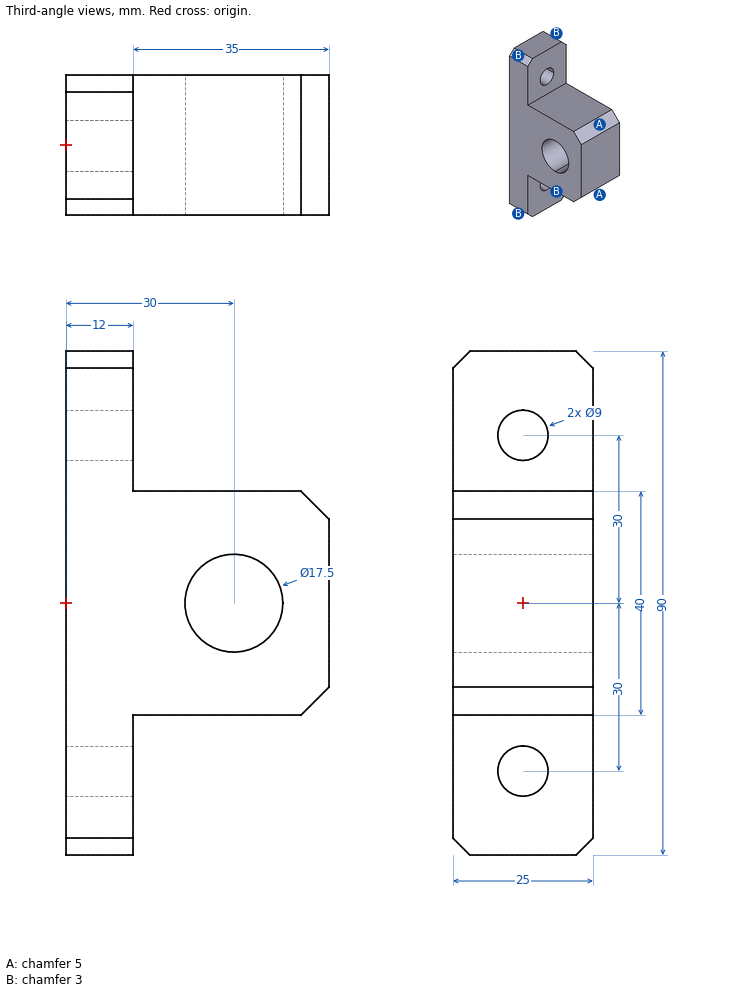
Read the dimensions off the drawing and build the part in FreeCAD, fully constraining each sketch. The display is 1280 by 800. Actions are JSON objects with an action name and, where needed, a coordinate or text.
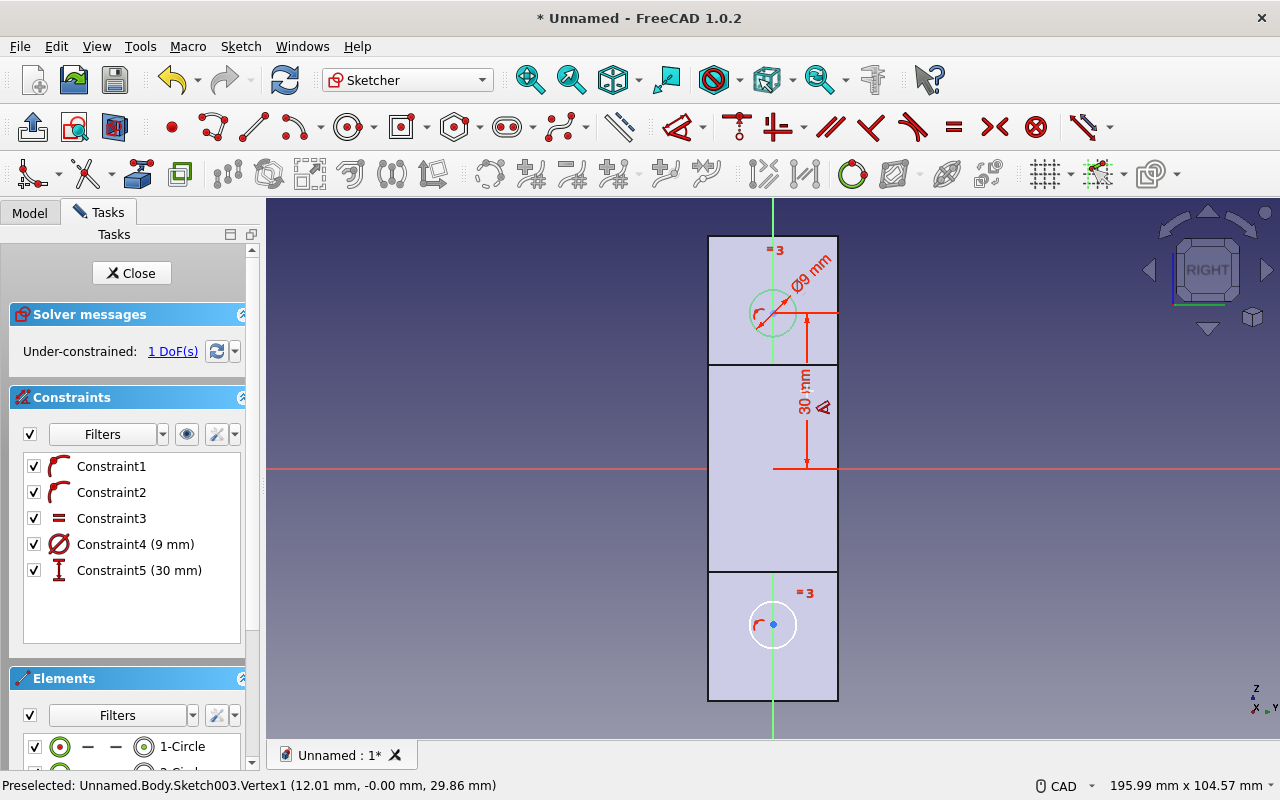
{"action": "left_click", "coordinate": [773, 625]}
{"action": "left_click", "coordinate": [807, 547]}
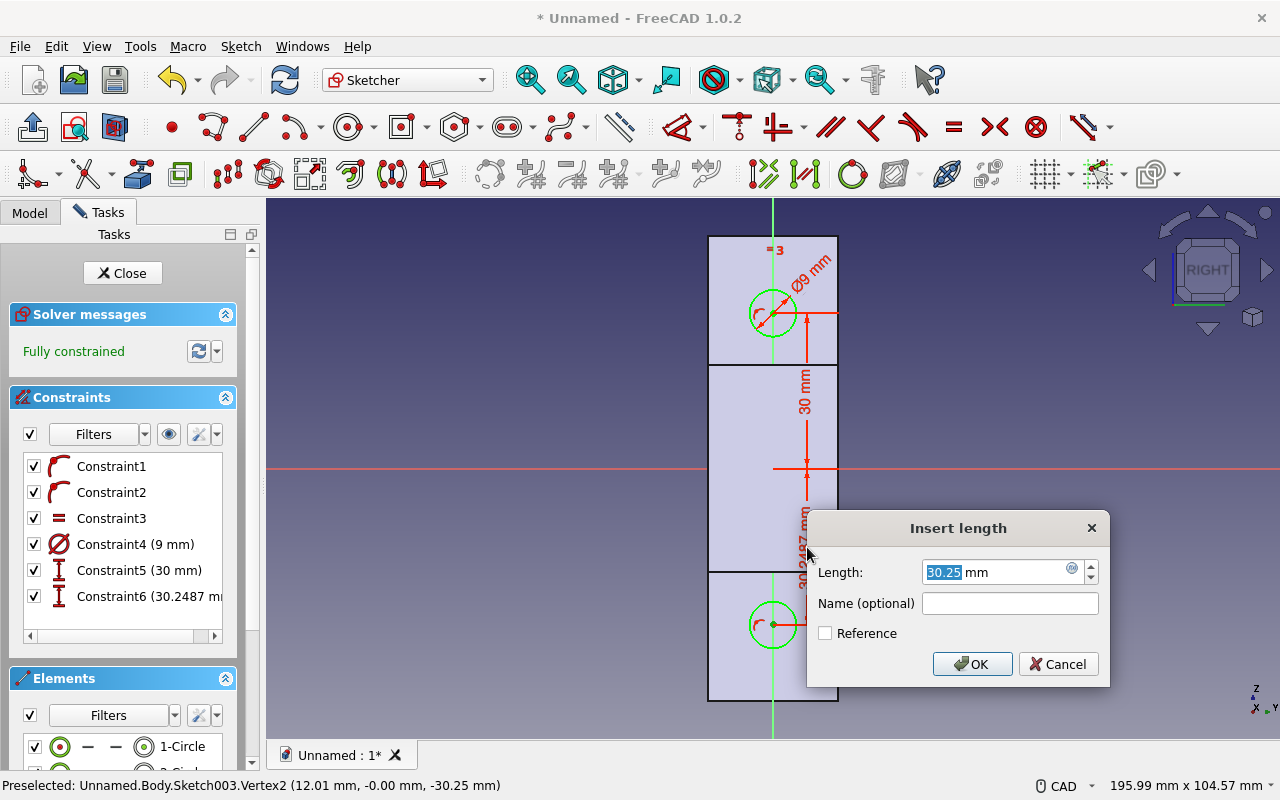
{"action": "type", "text": "30"}
{"action": "key", "text": "Return"}
{"action": "key", "text": "Escape"}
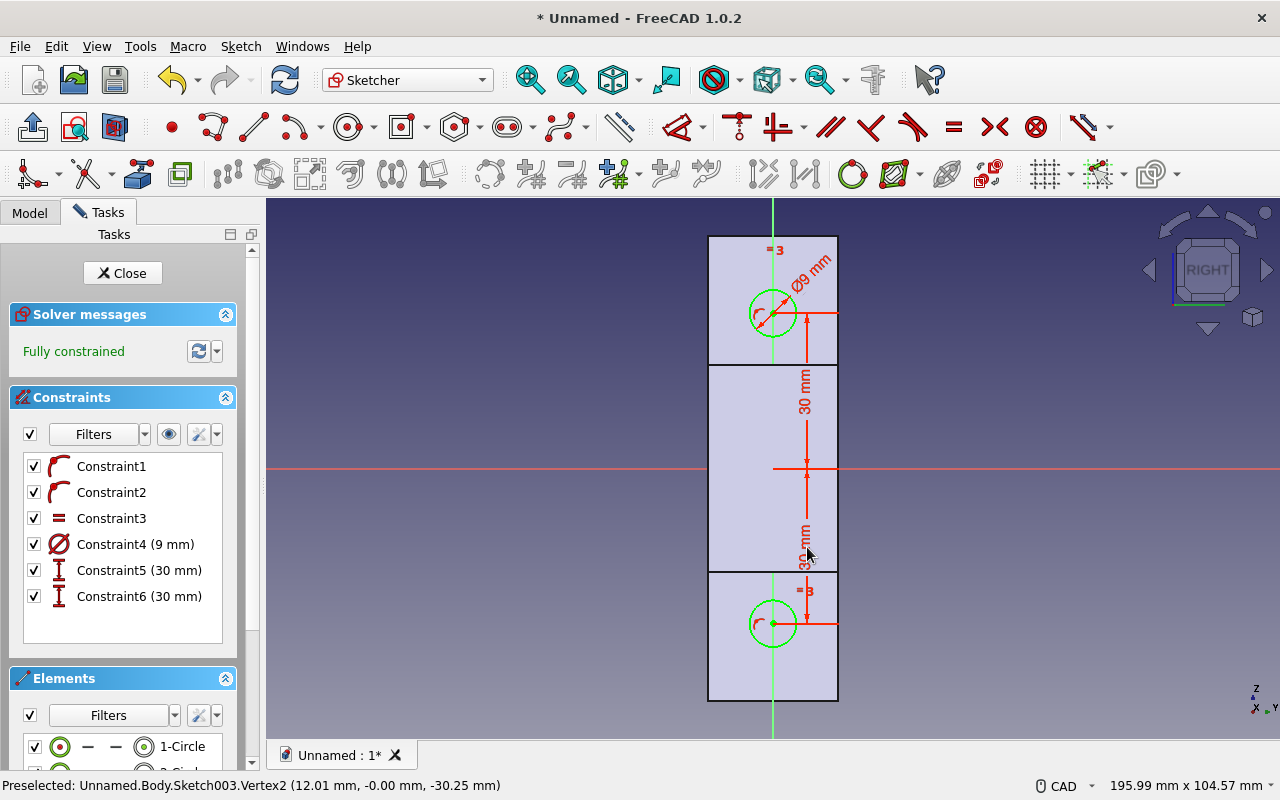
{"action": "left_click", "coordinate": [123, 273]}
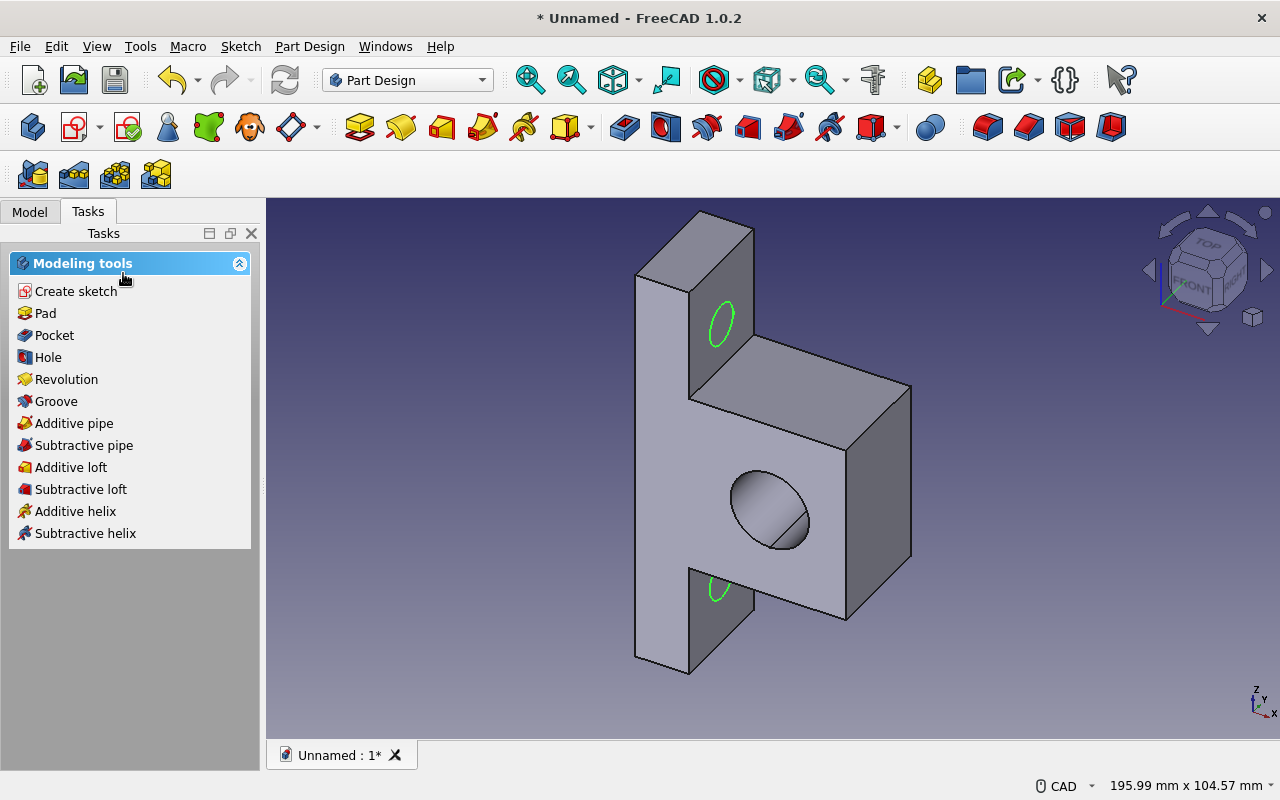
{"action": "left_click", "coordinate": [625, 128]}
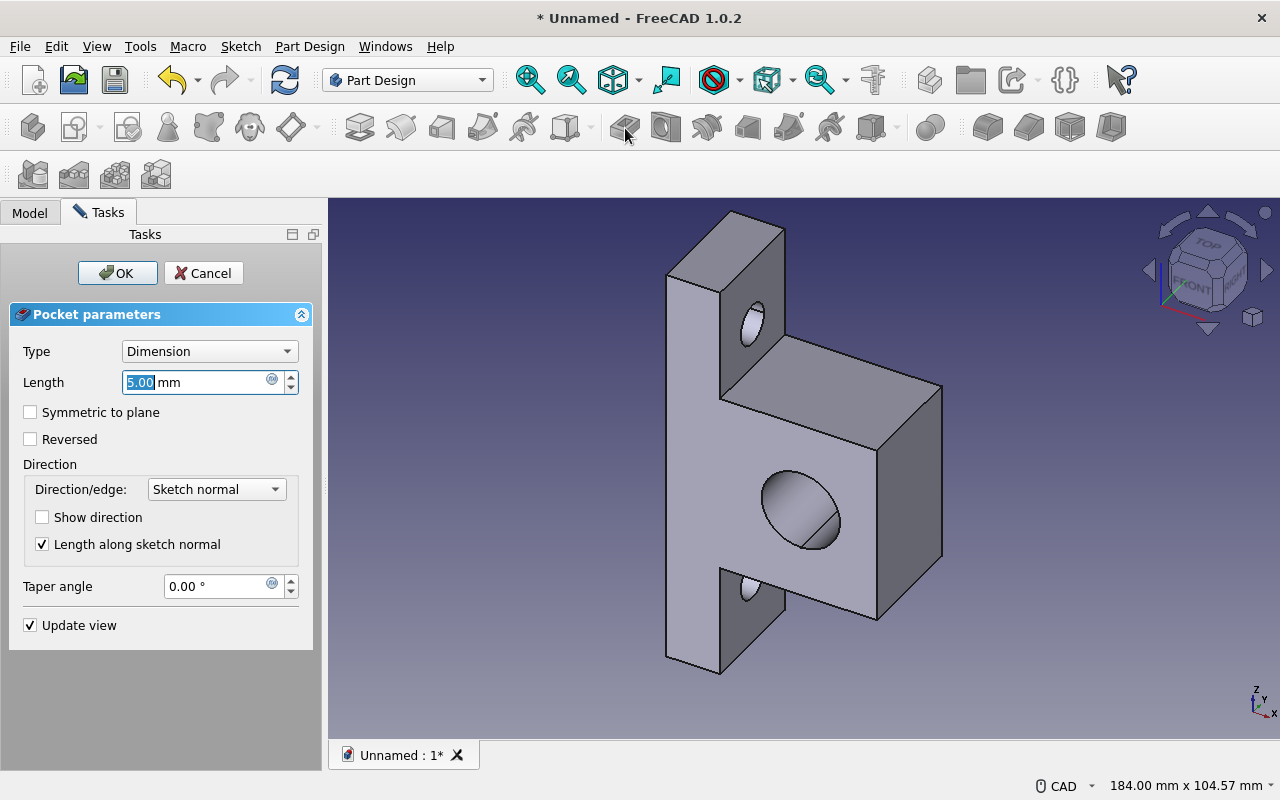
{"action": "left_click", "coordinate": [210, 352]}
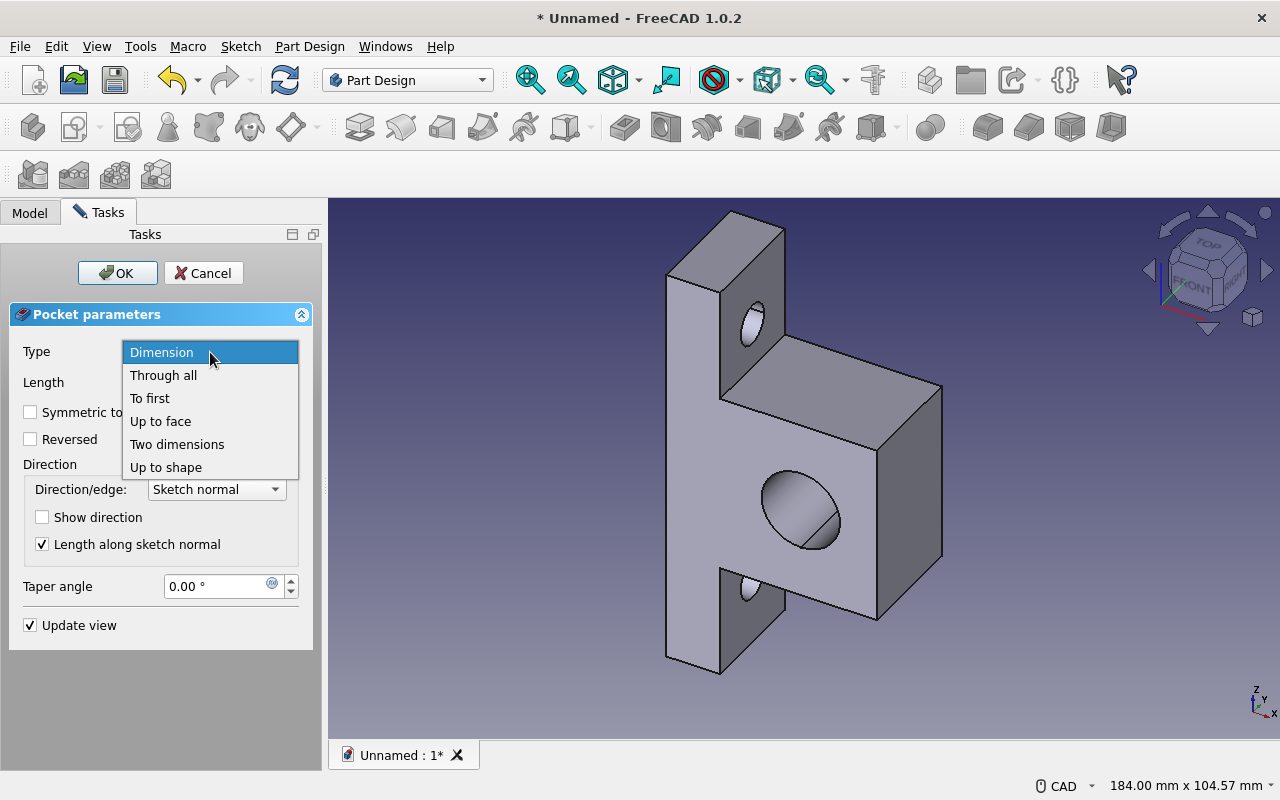
{"action": "left_click", "coordinate": [208, 376]}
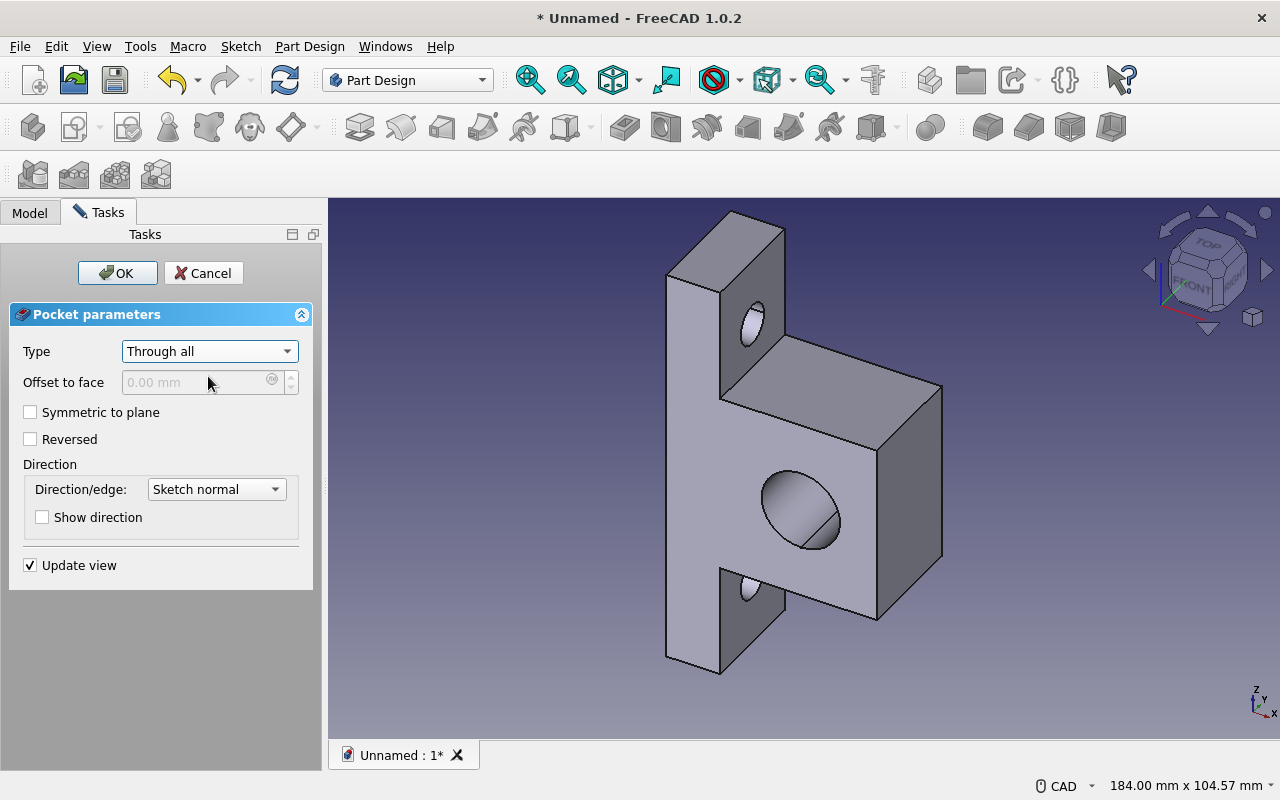
{"action": "left_click", "coordinate": [118, 273]}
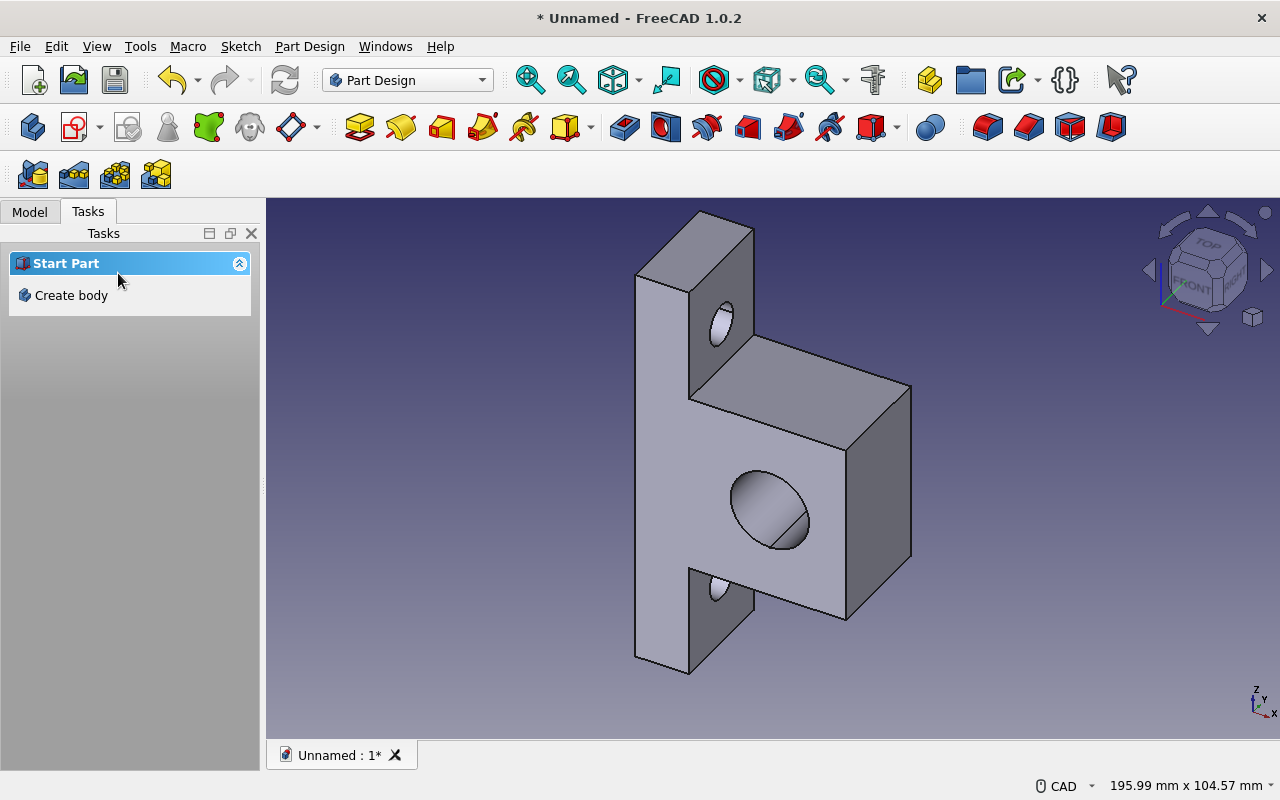
{"action": "left_click", "coordinate": [878, 418]}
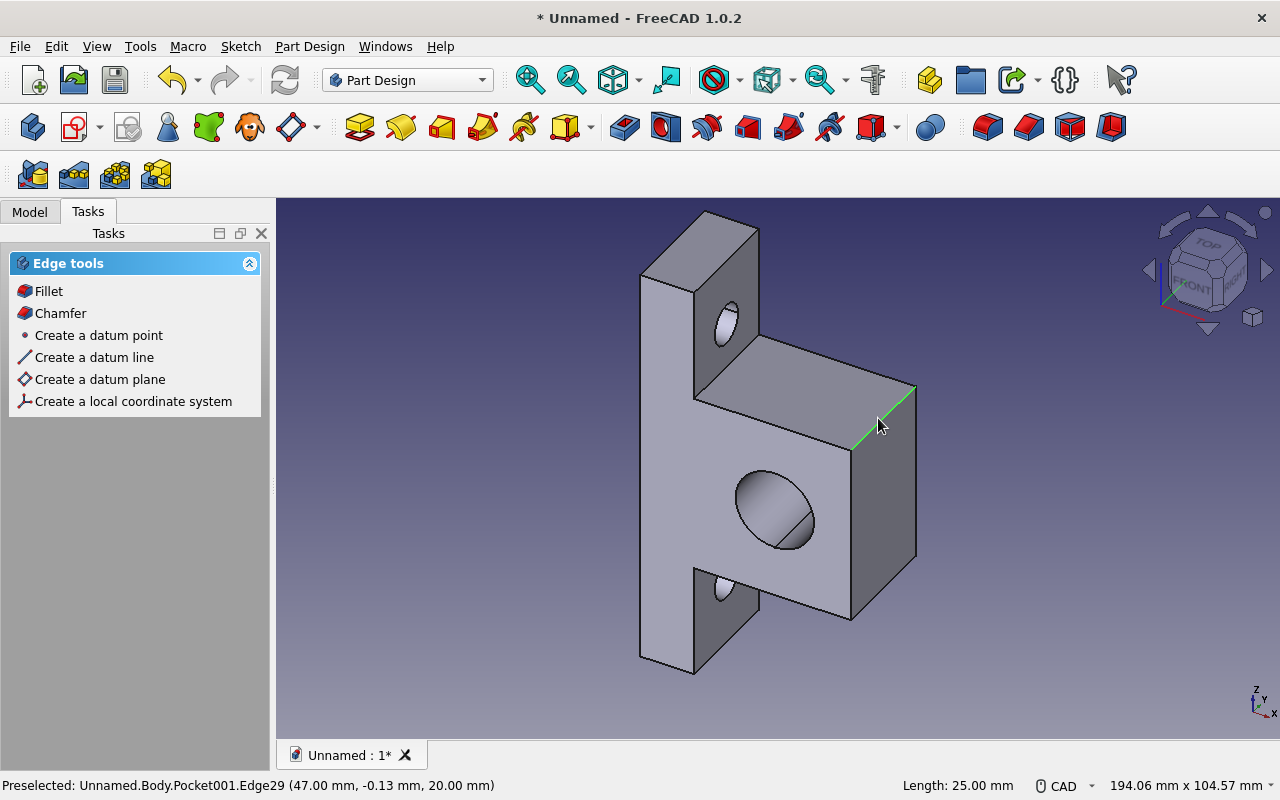
{"action": "key", "text": "0"}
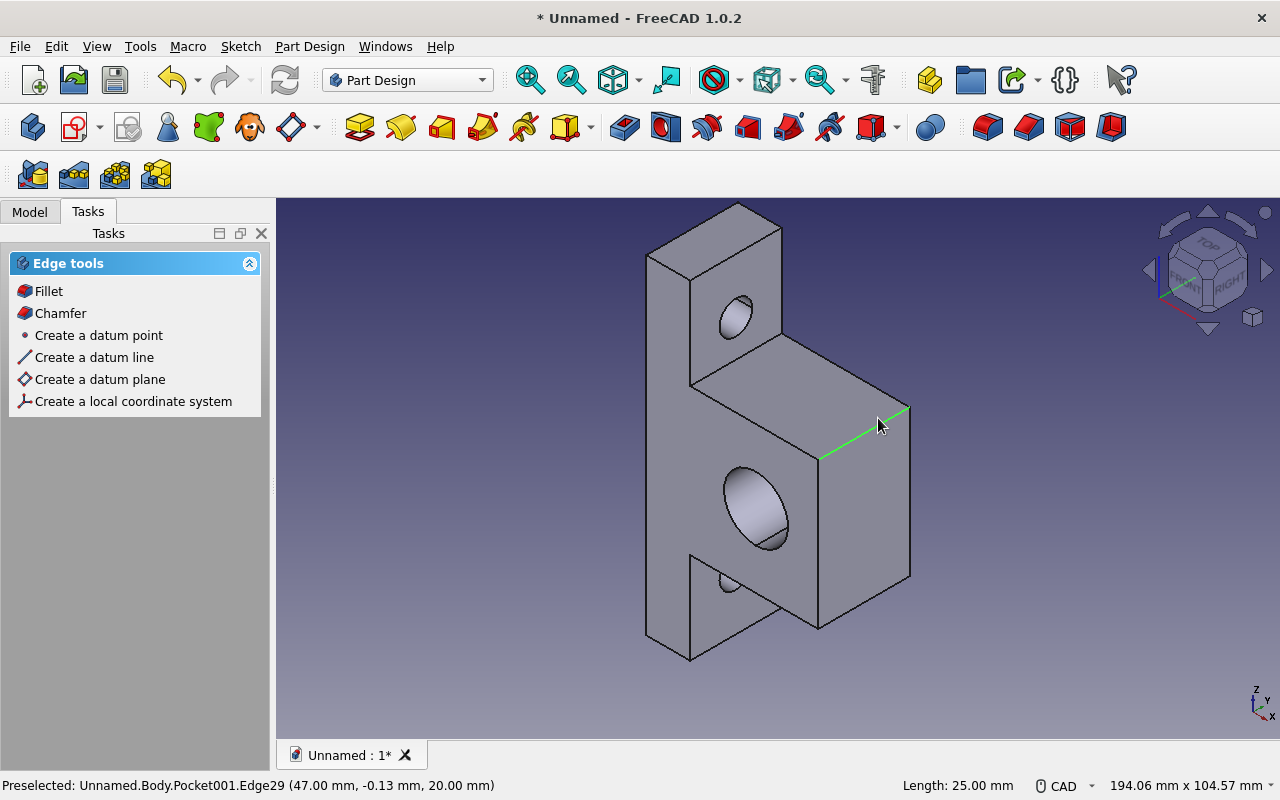
{"action": "key", "text": "2"}